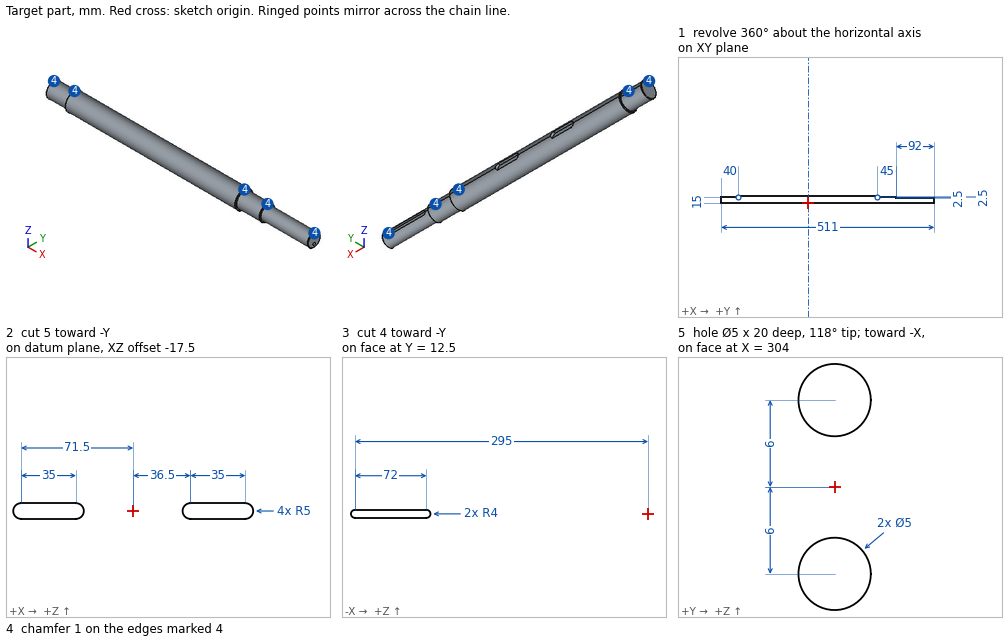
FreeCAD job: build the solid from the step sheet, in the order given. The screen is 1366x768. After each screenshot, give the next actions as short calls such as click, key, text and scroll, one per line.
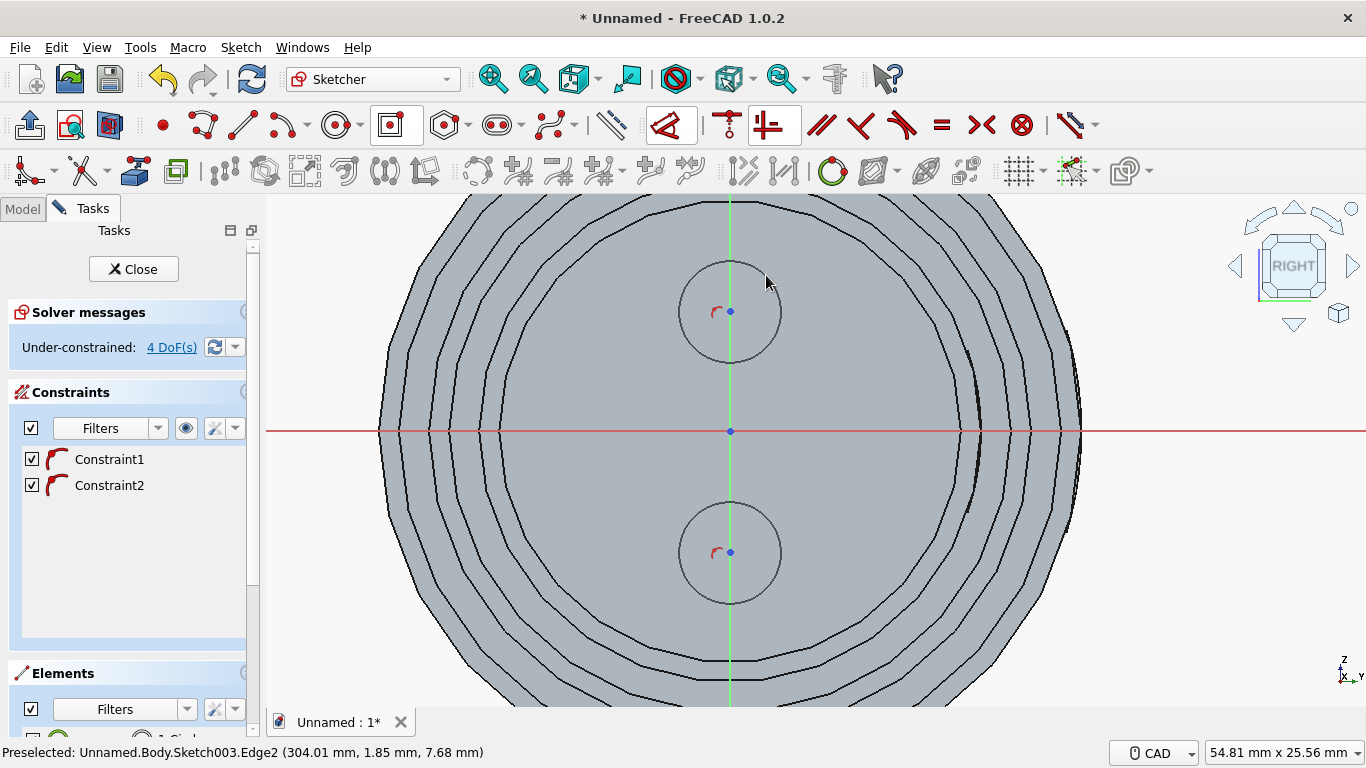
click(766, 517)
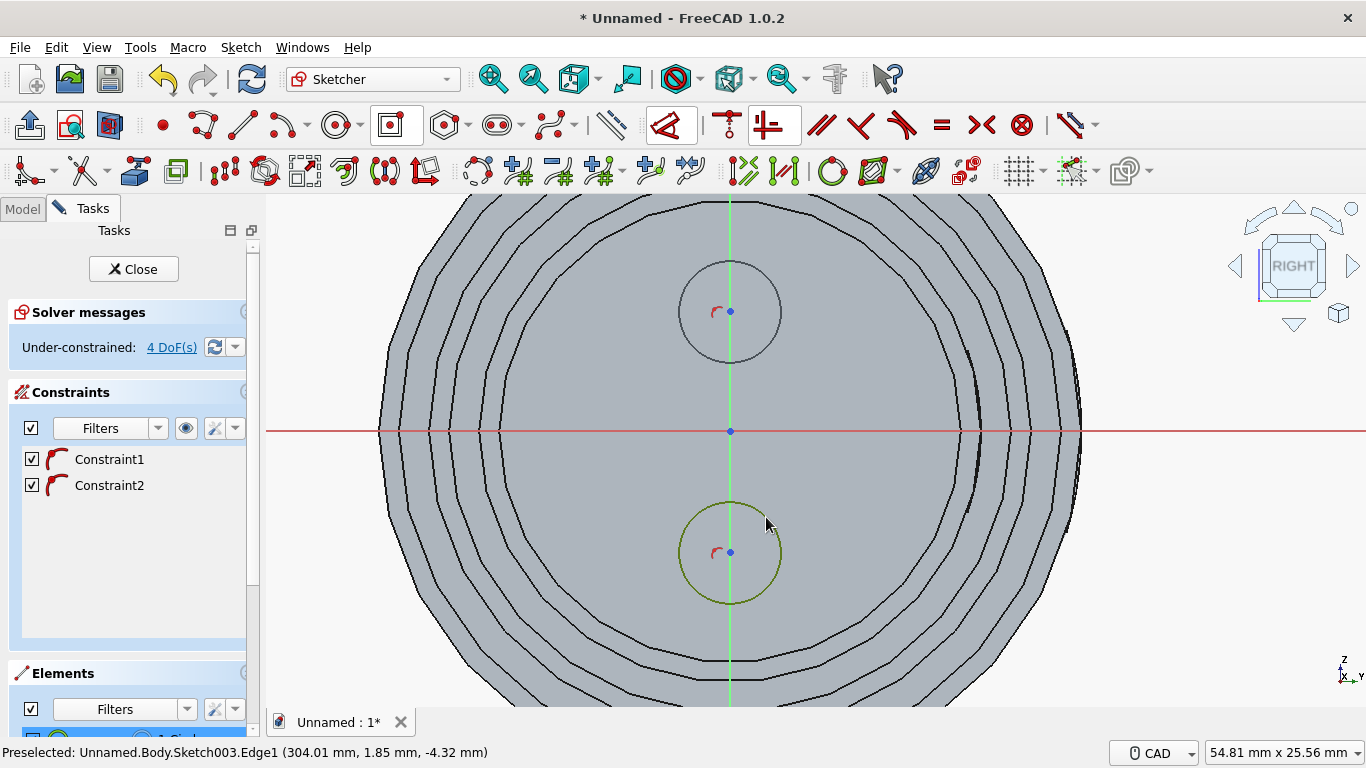
click(766, 276)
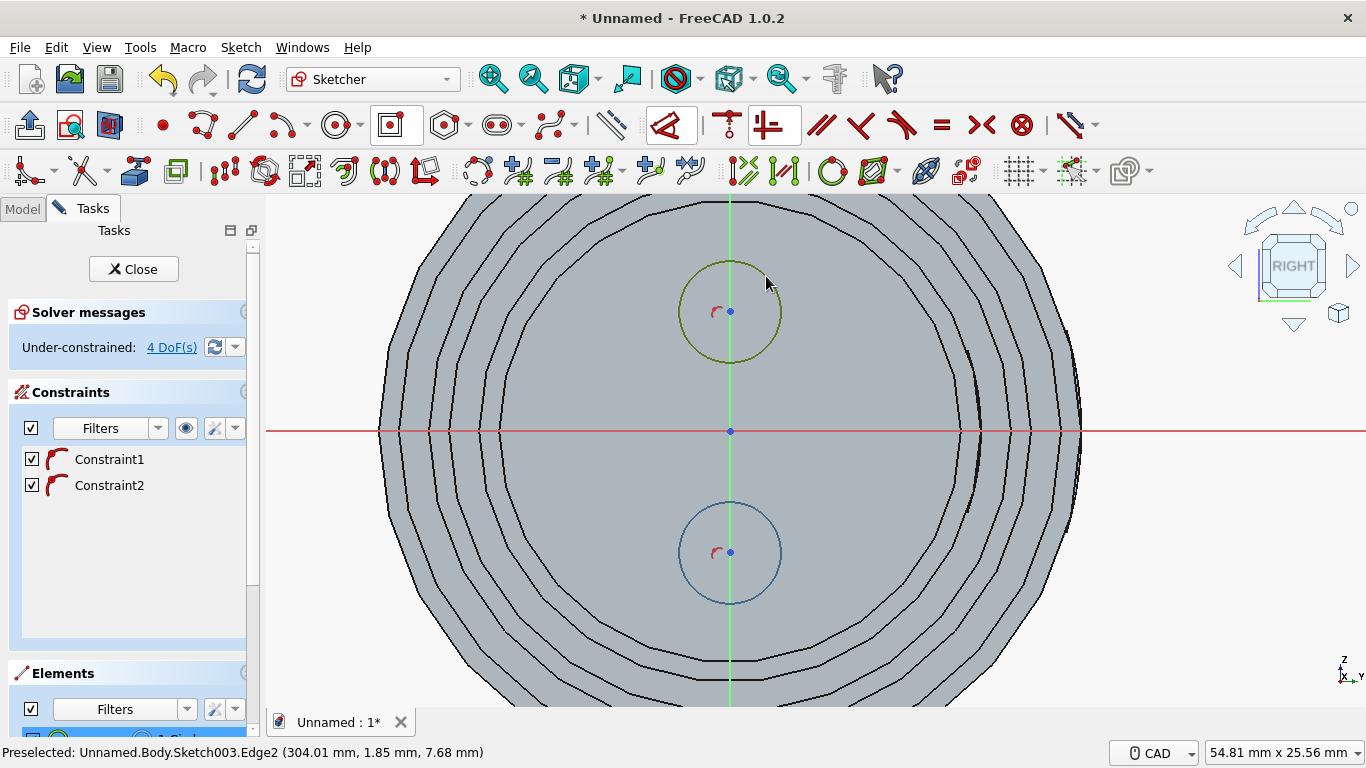
key(e)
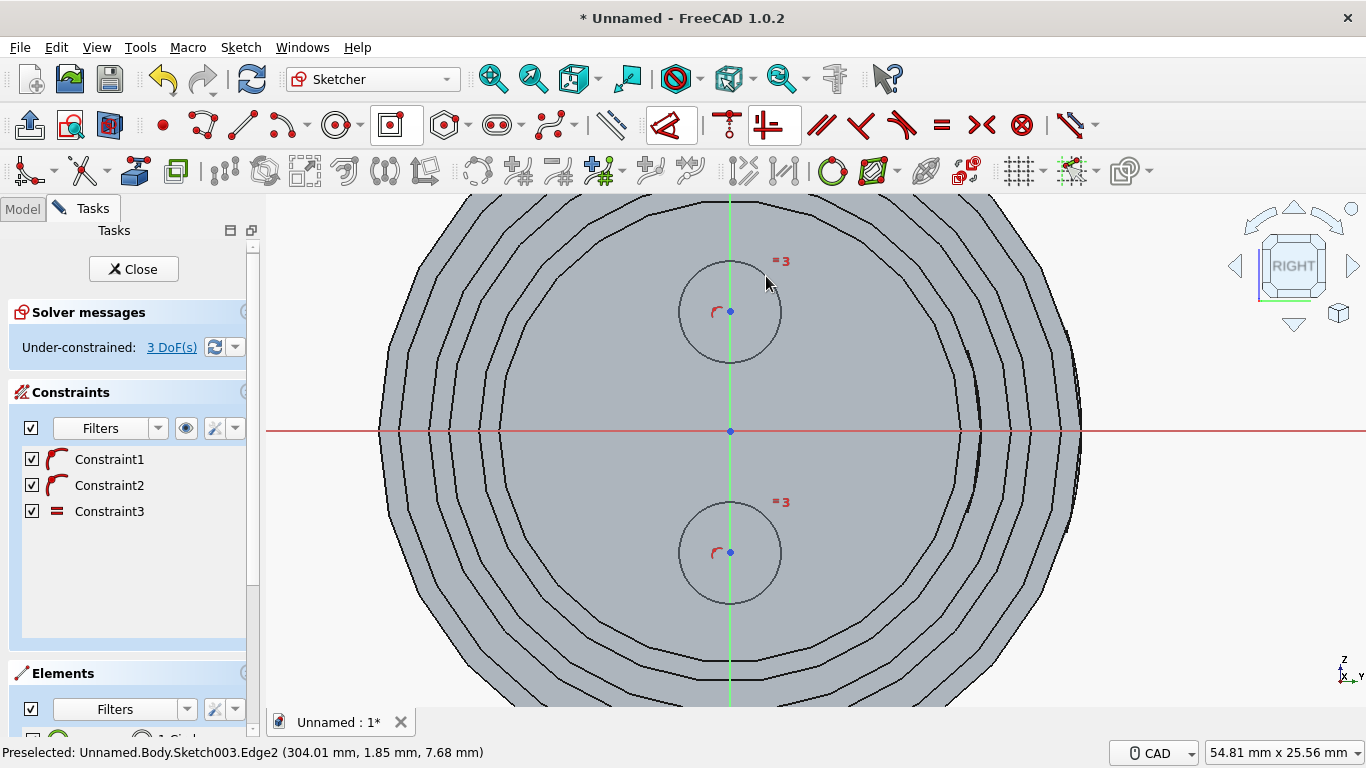
click(766, 517)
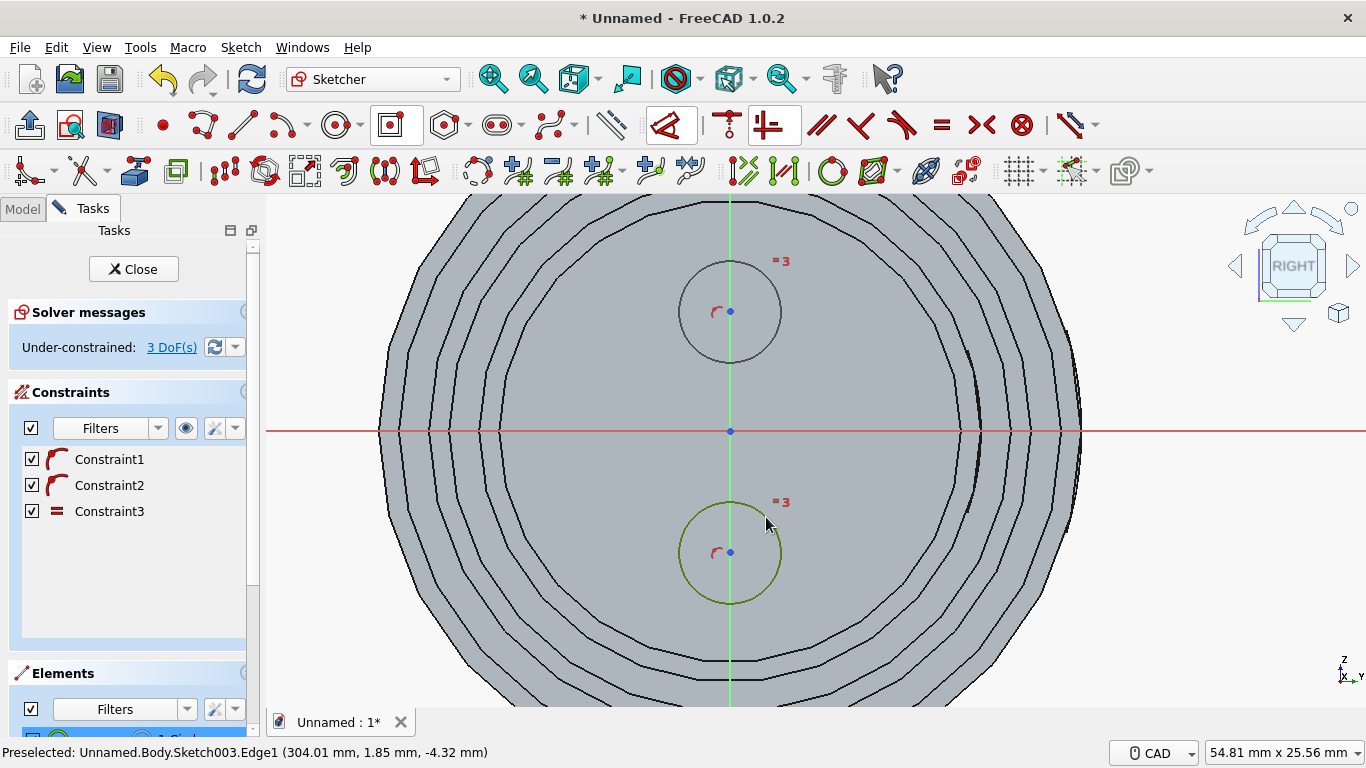
click(692, 126)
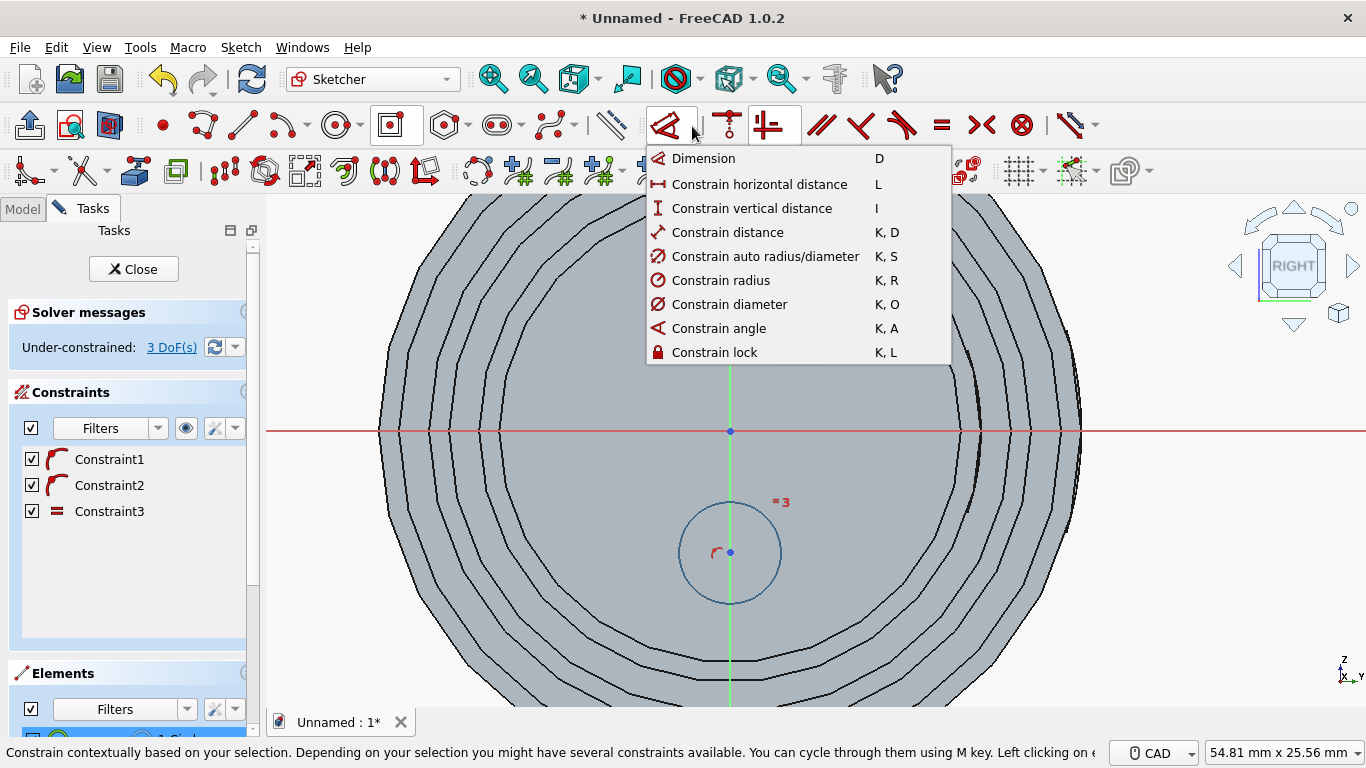
click(799, 304)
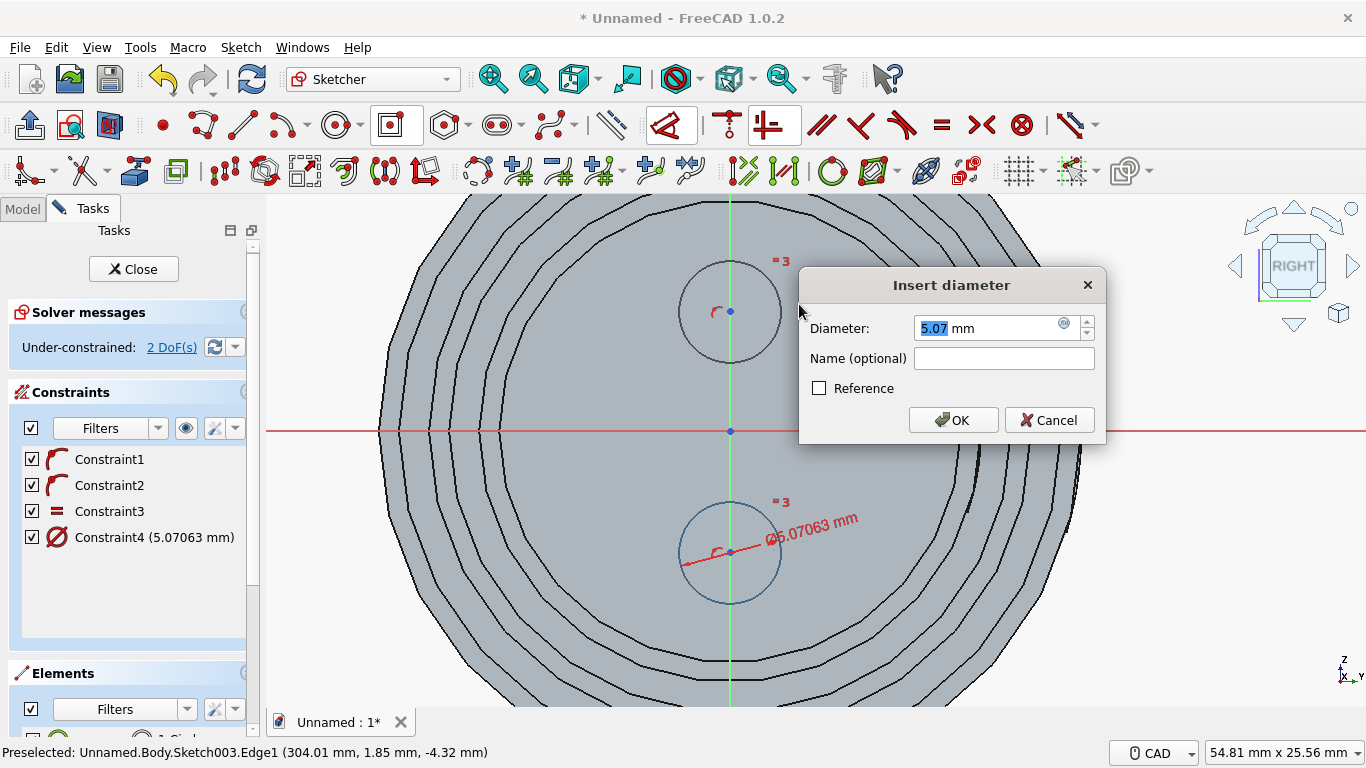
text(5)
key(Return)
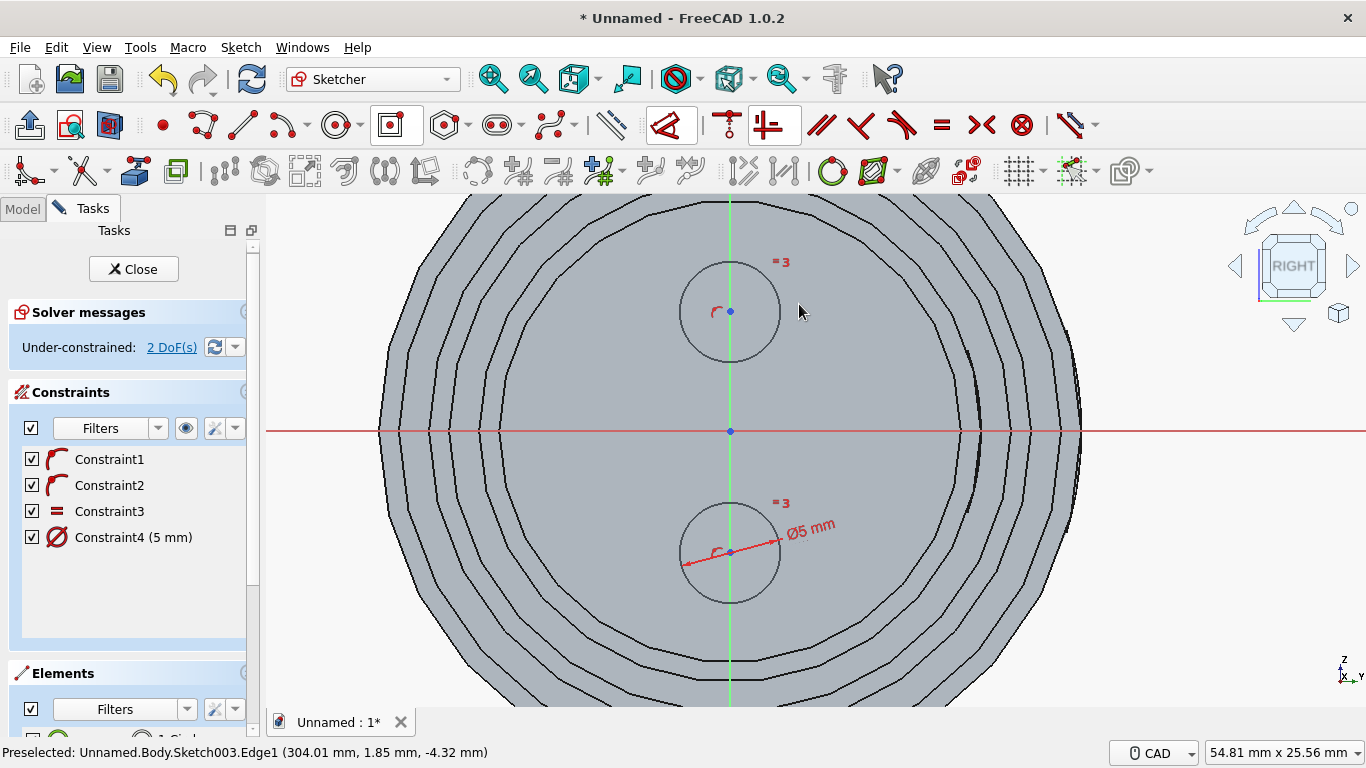
click(730, 553)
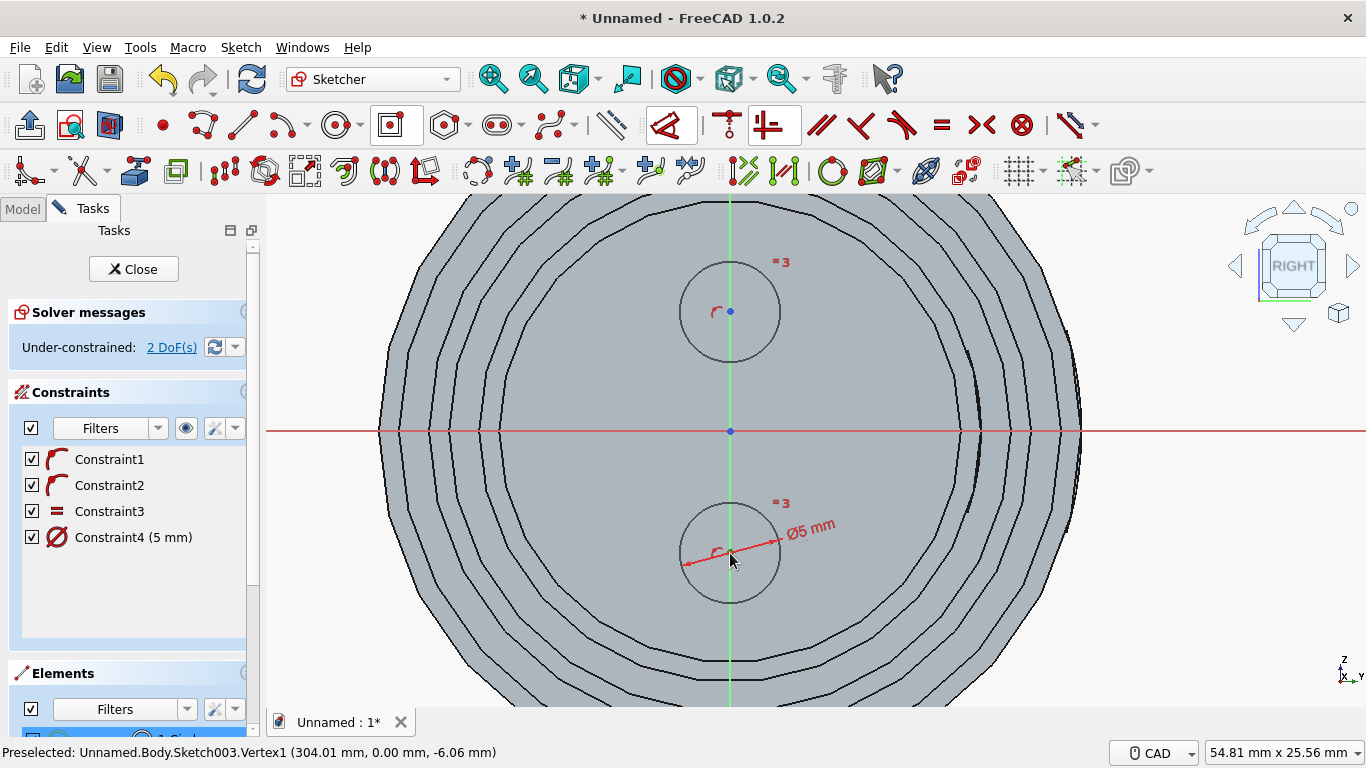
click(692, 126)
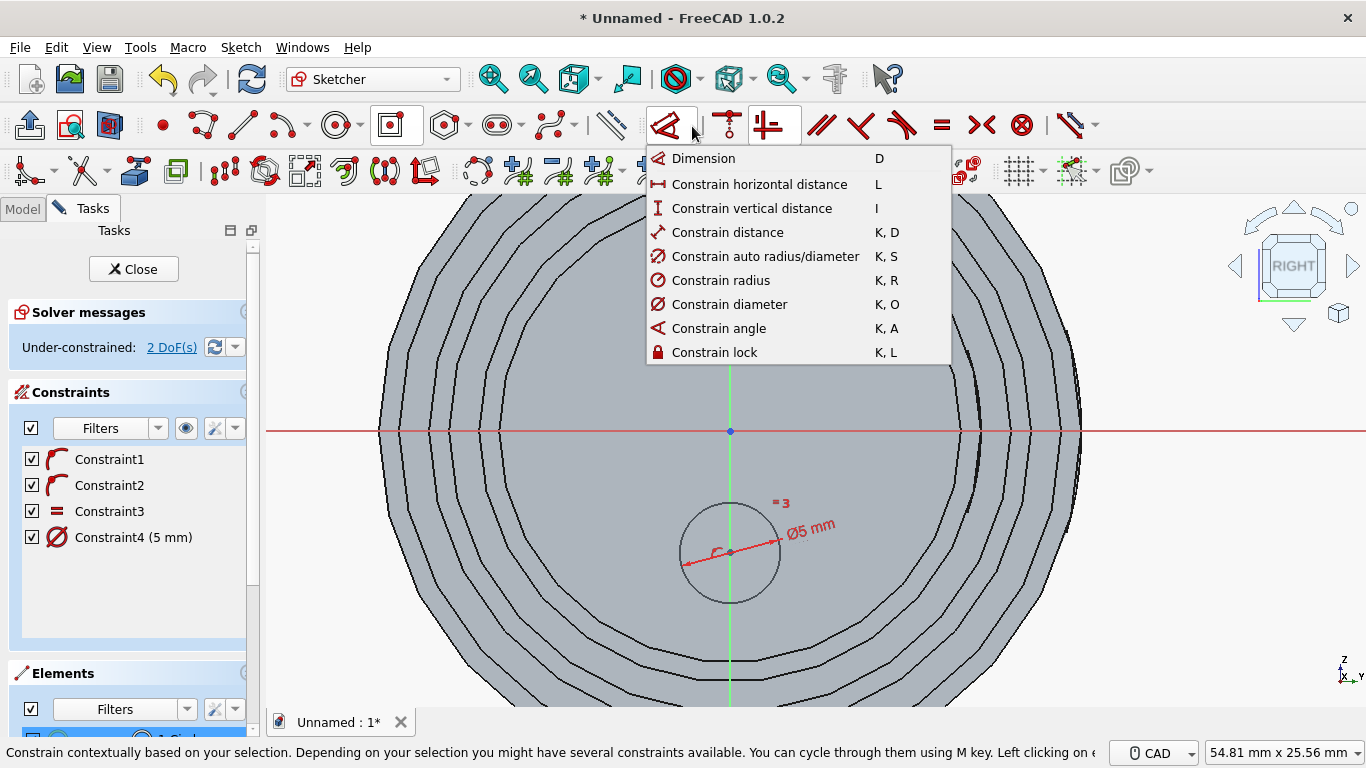
click(799, 208)